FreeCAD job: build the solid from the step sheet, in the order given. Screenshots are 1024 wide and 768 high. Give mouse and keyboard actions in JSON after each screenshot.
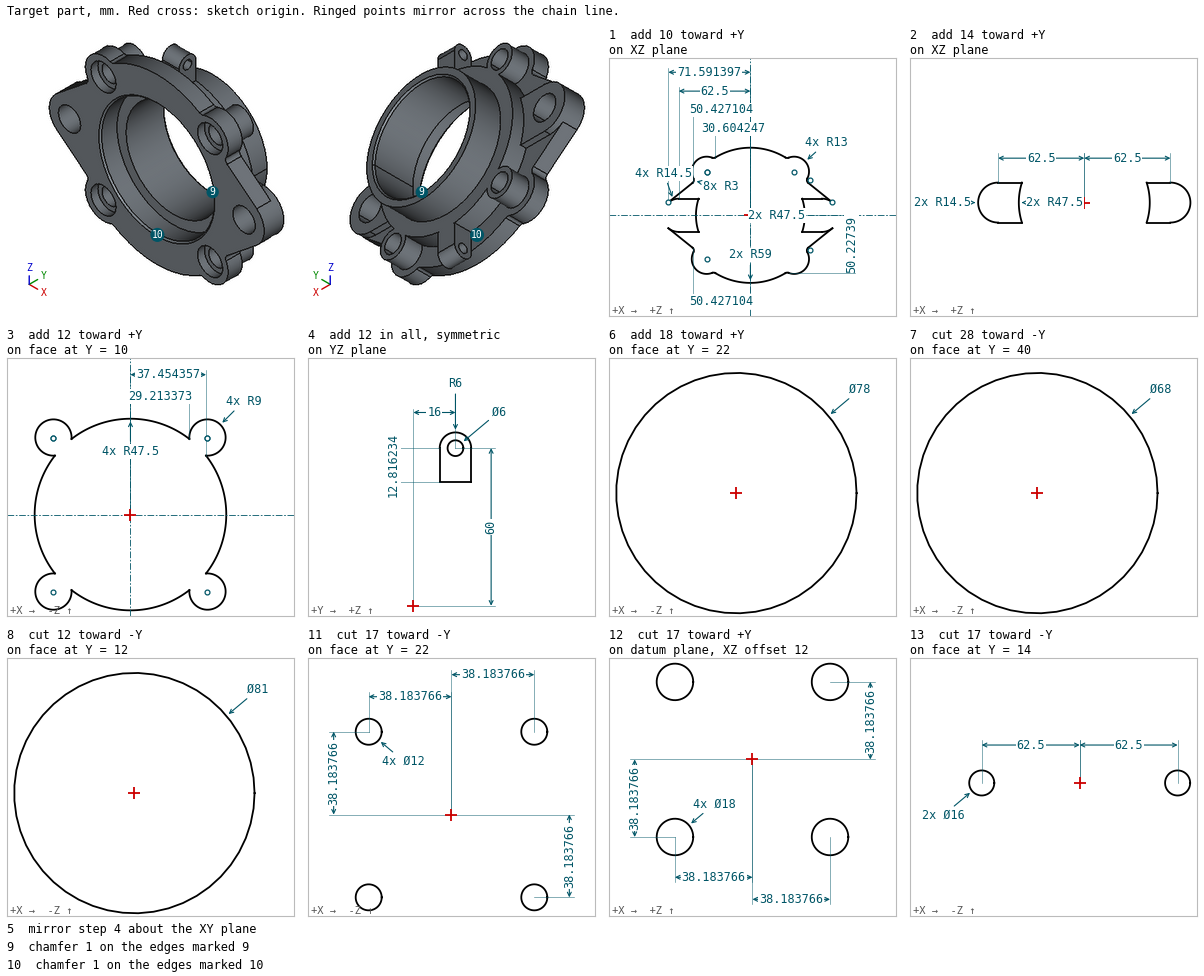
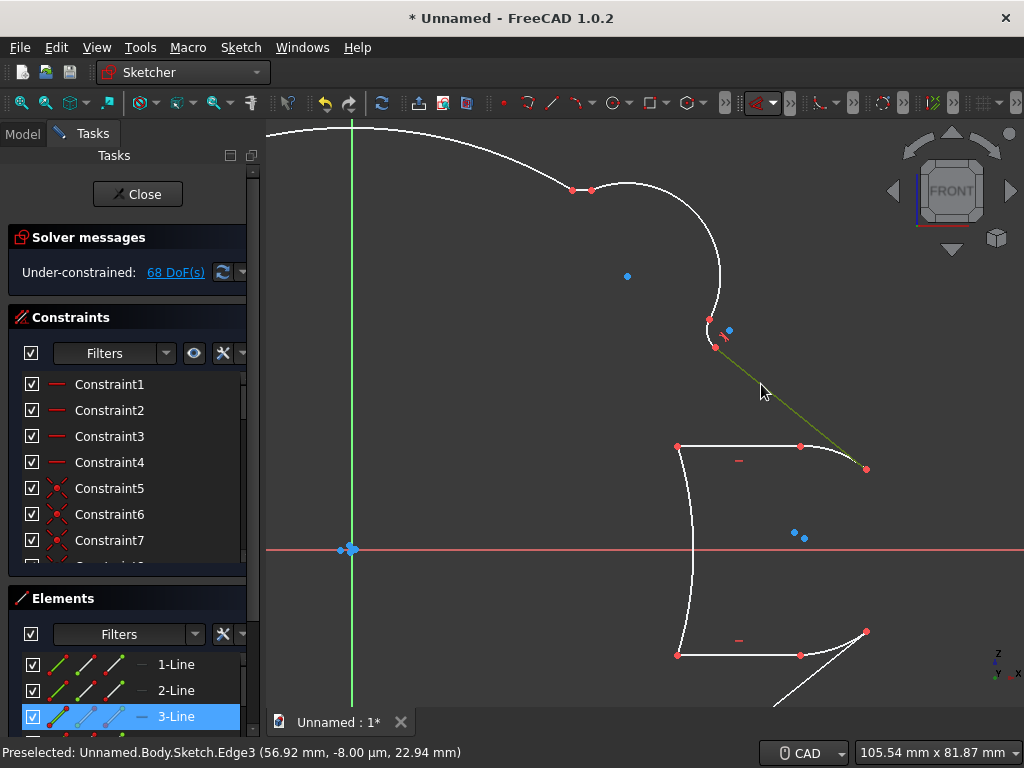
{"action": "scroll", "coordinate": [822, 448], "scroll_direction": "up", "scroll_amount": 2}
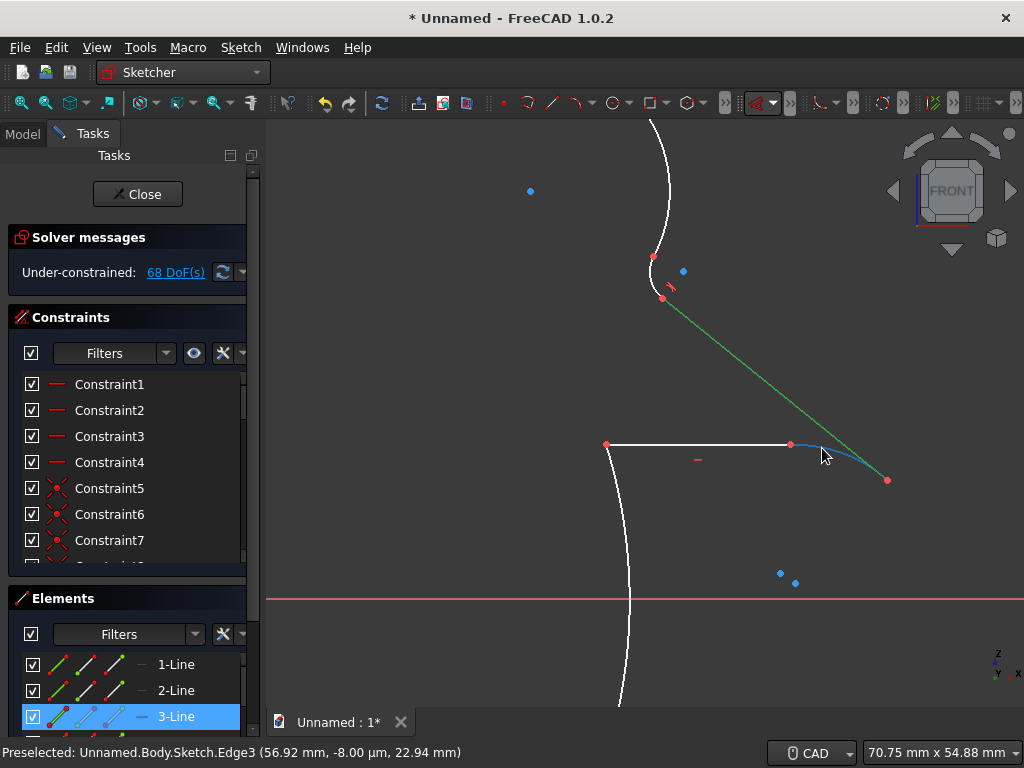
{"action": "left_click", "coordinate": [822, 447]}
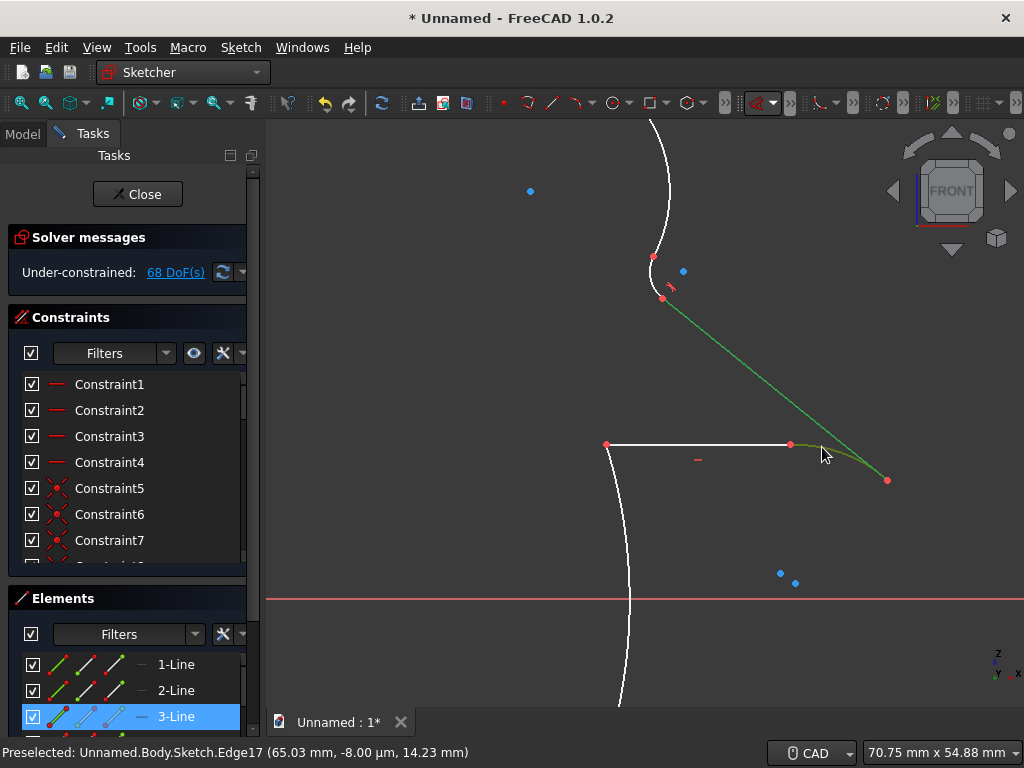
{"action": "key", "text": "t"}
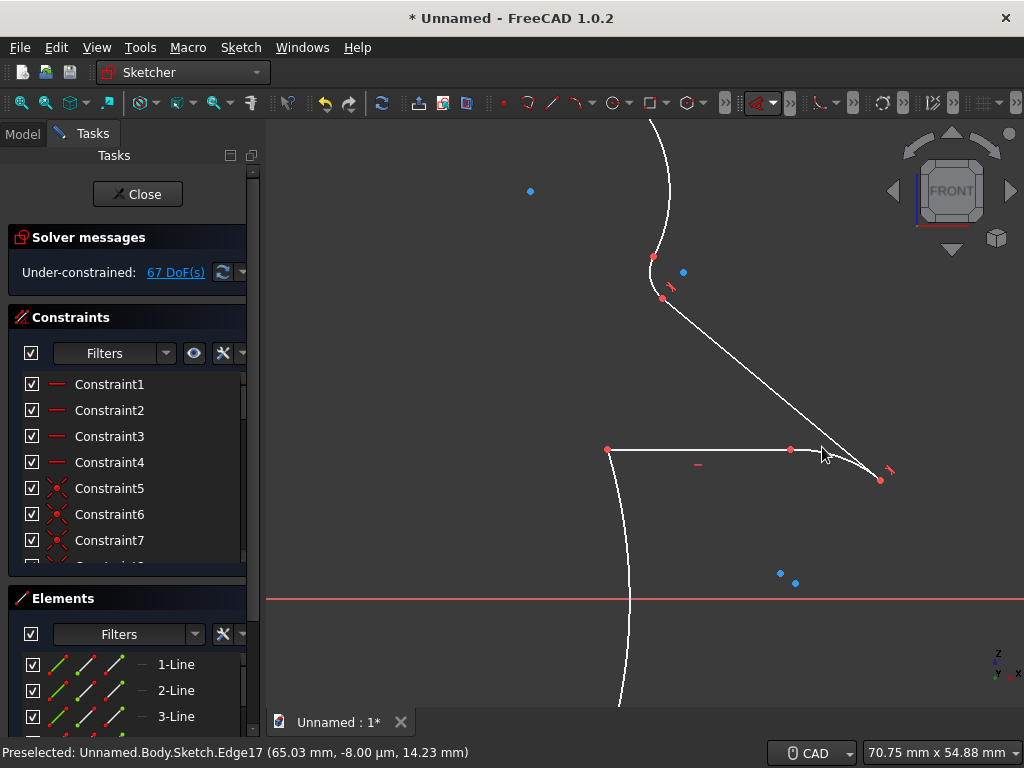
{"action": "scroll", "coordinate": [726, 352], "scroll_direction": "down", "scroll_amount": 7}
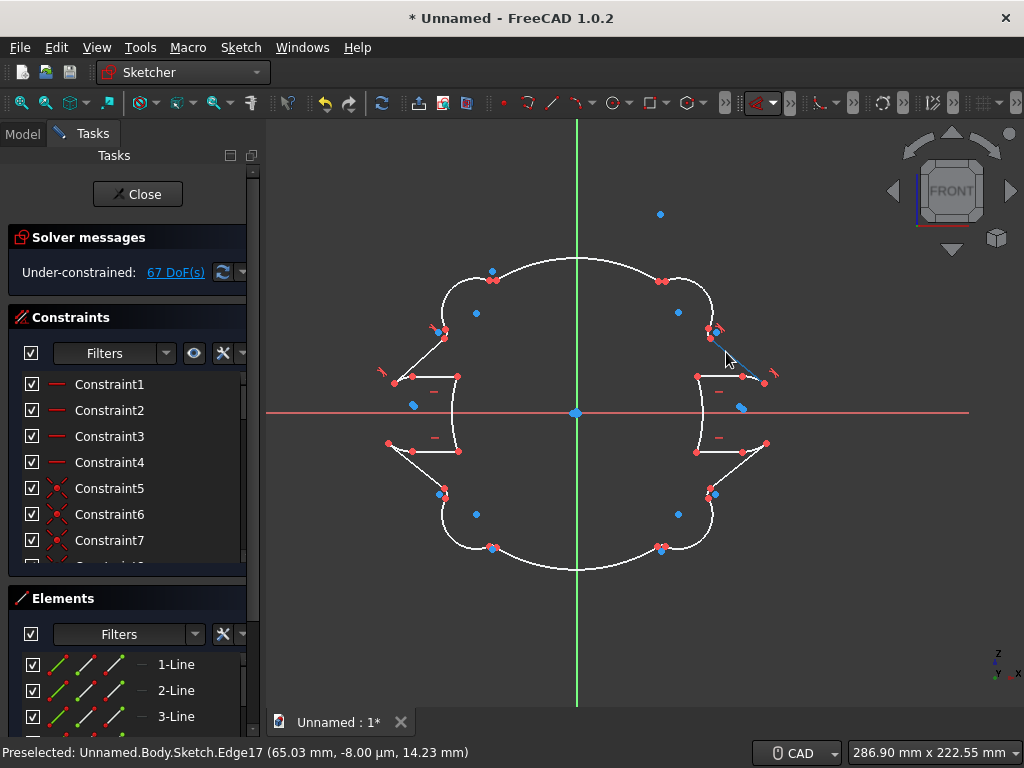
{"action": "left_click", "coordinate": [729, 376]}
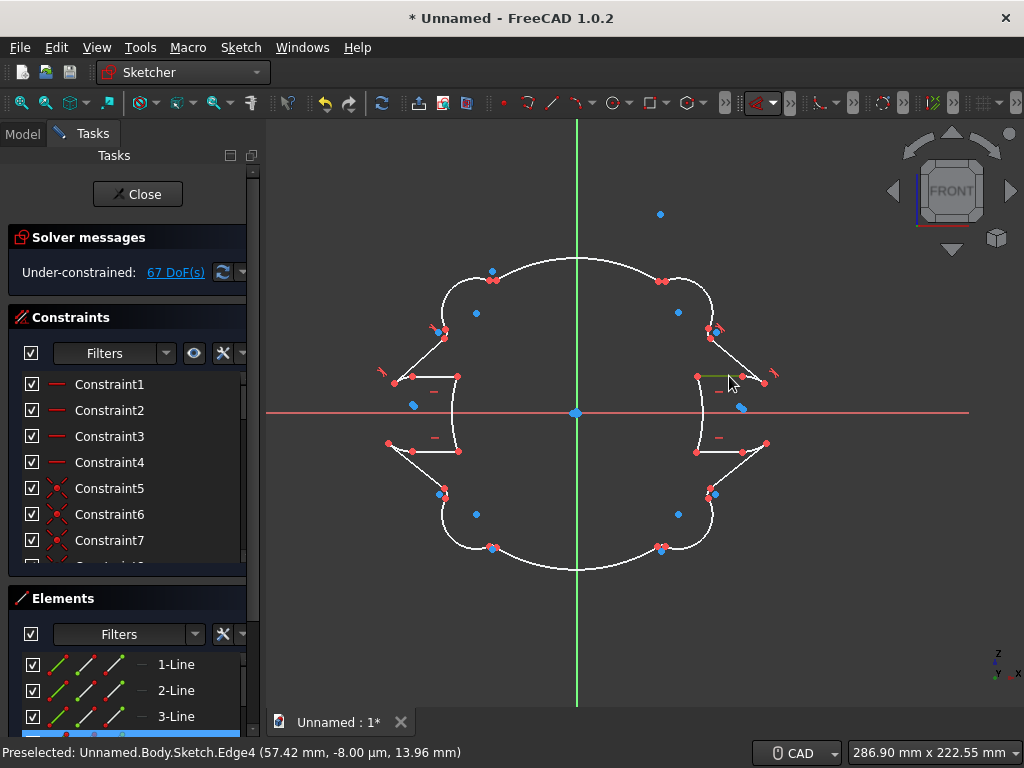
{"action": "scroll", "coordinate": [747, 377], "scroll_direction": "up", "scroll_amount": 6}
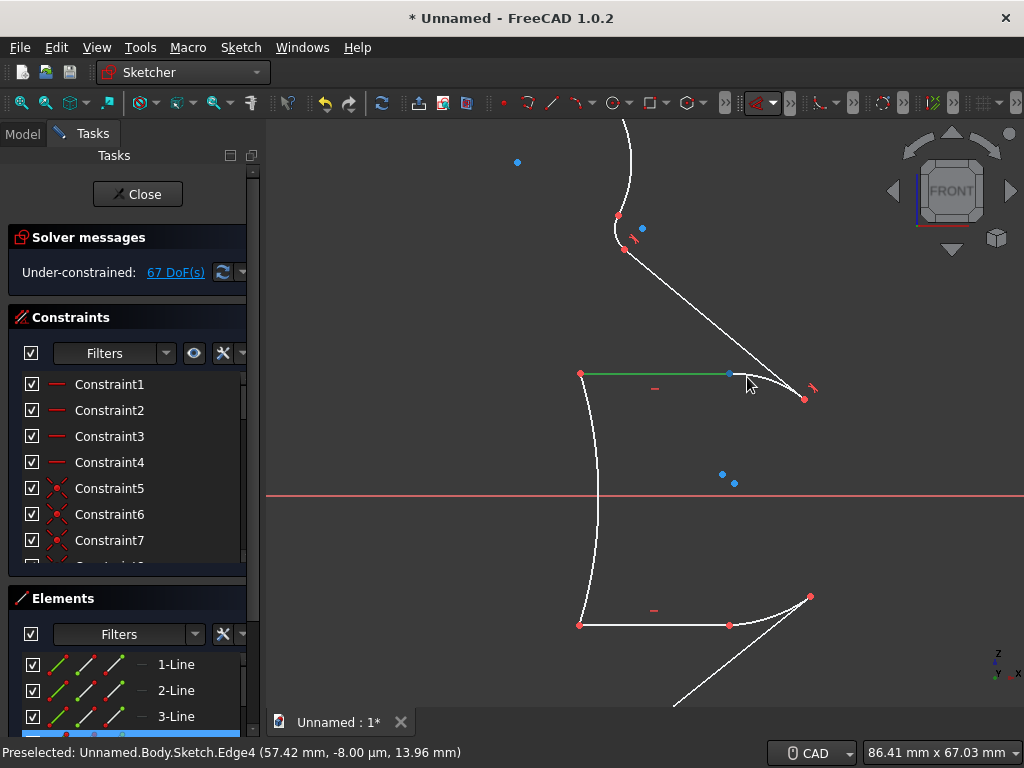
{"action": "left_click", "coordinate": [746, 374]}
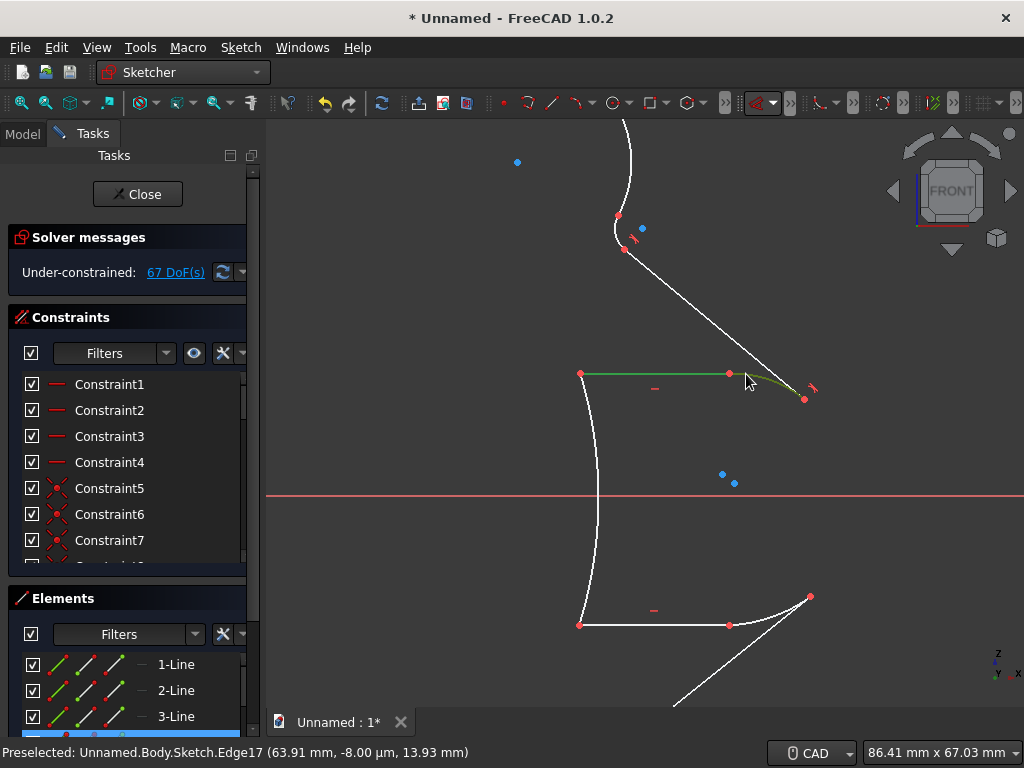
{"action": "key", "text": "t"}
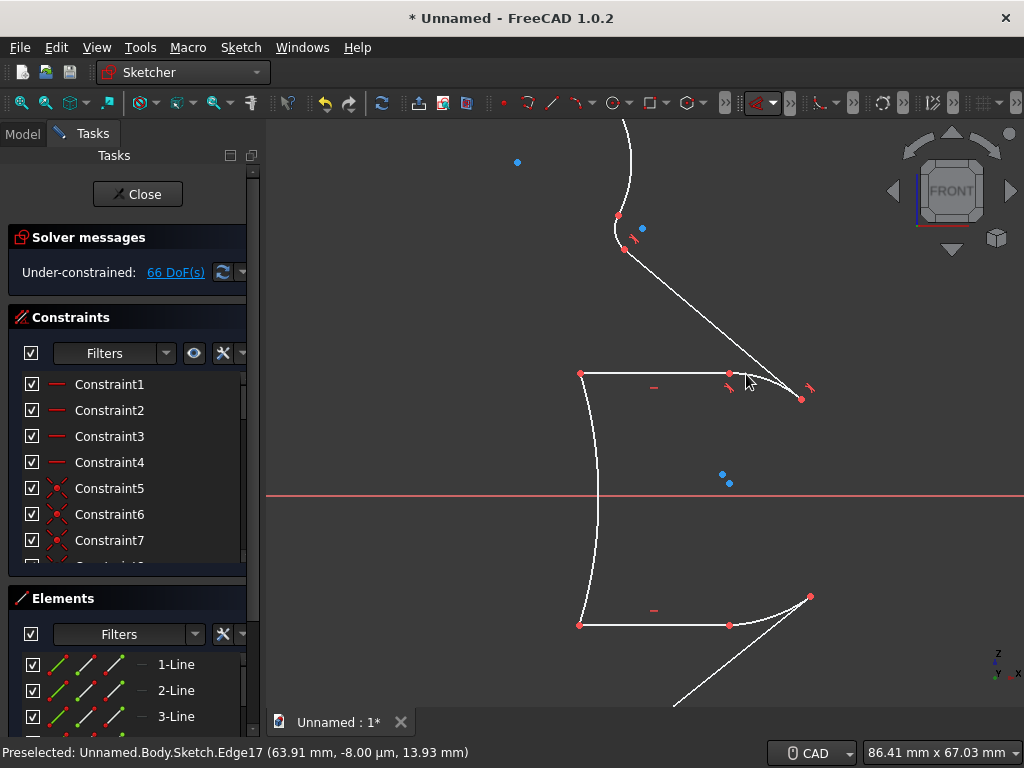
{"action": "left_click", "coordinate": [624, 625]}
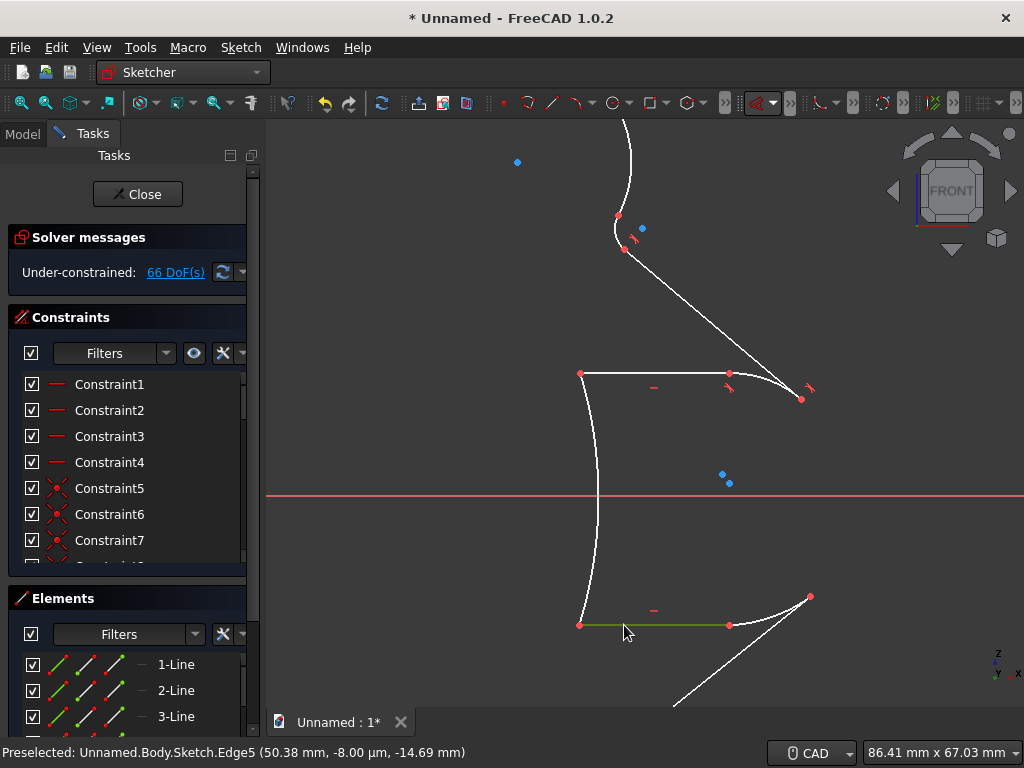
{"action": "left_click", "coordinate": [756, 622]}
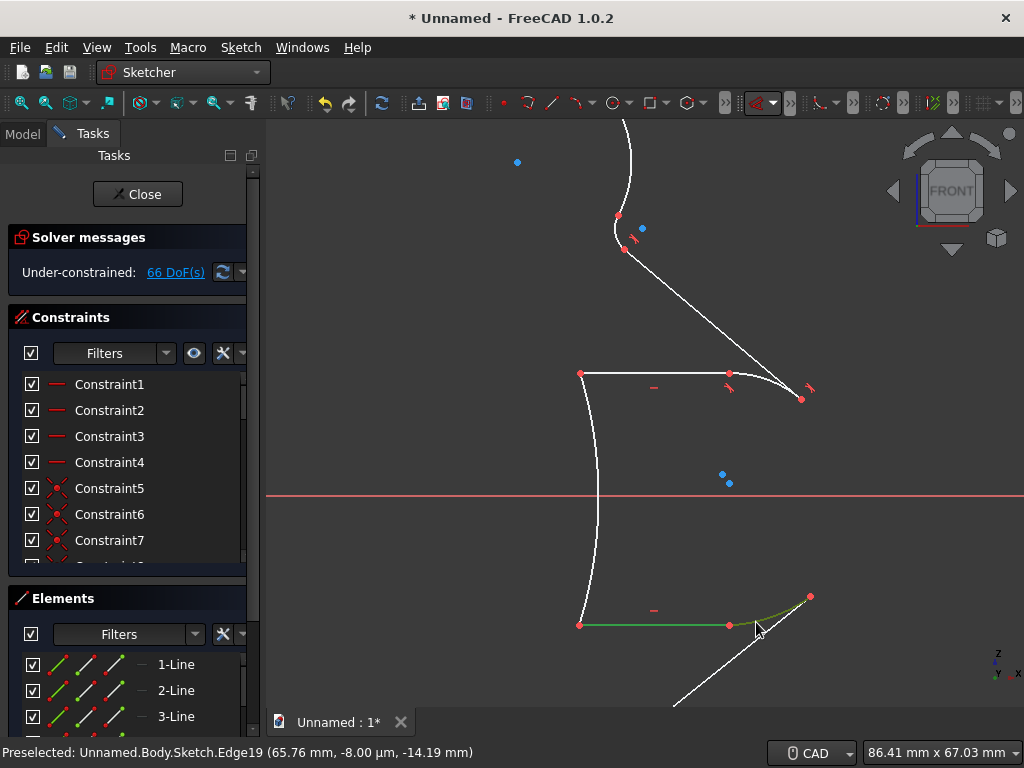
{"action": "key", "text": "t"}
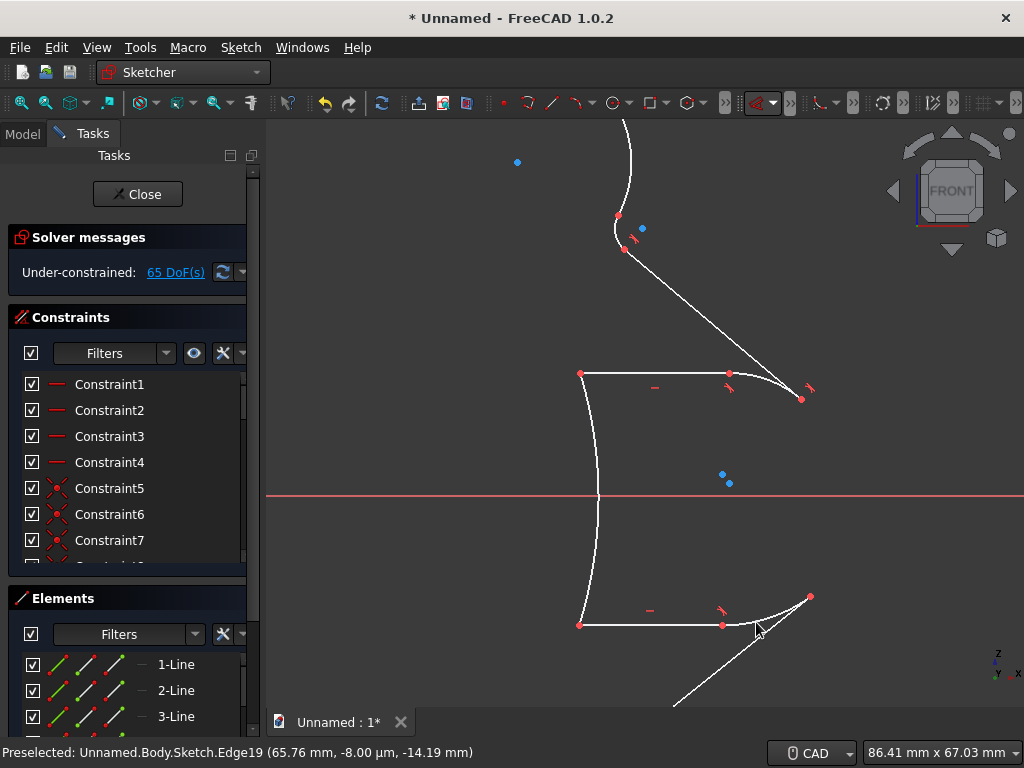
{"action": "left_click", "coordinate": [754, 642]}